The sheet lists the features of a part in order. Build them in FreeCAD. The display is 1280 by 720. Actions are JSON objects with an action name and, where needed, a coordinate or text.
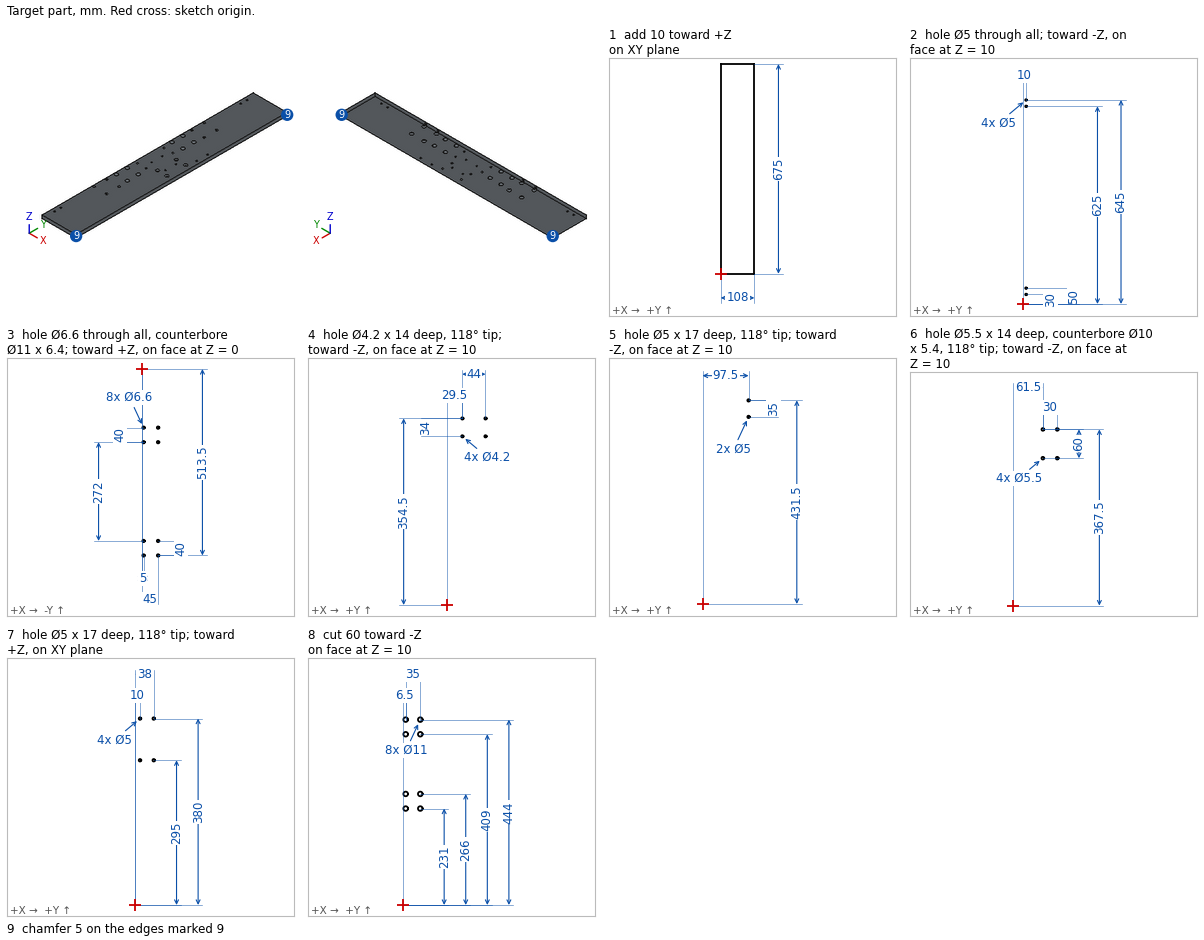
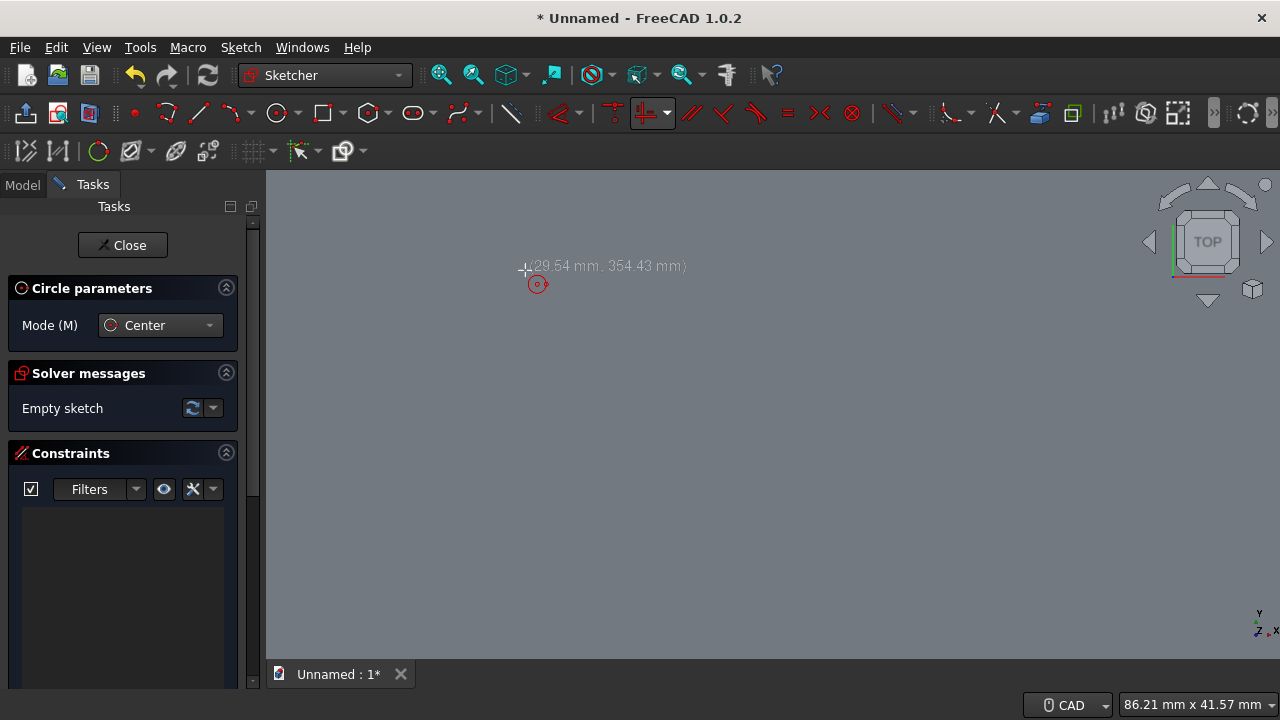
{"action": "left_click", "coordinate": [524, 271]}
{"action": "mouse_move", "coordinate": [542, 253]}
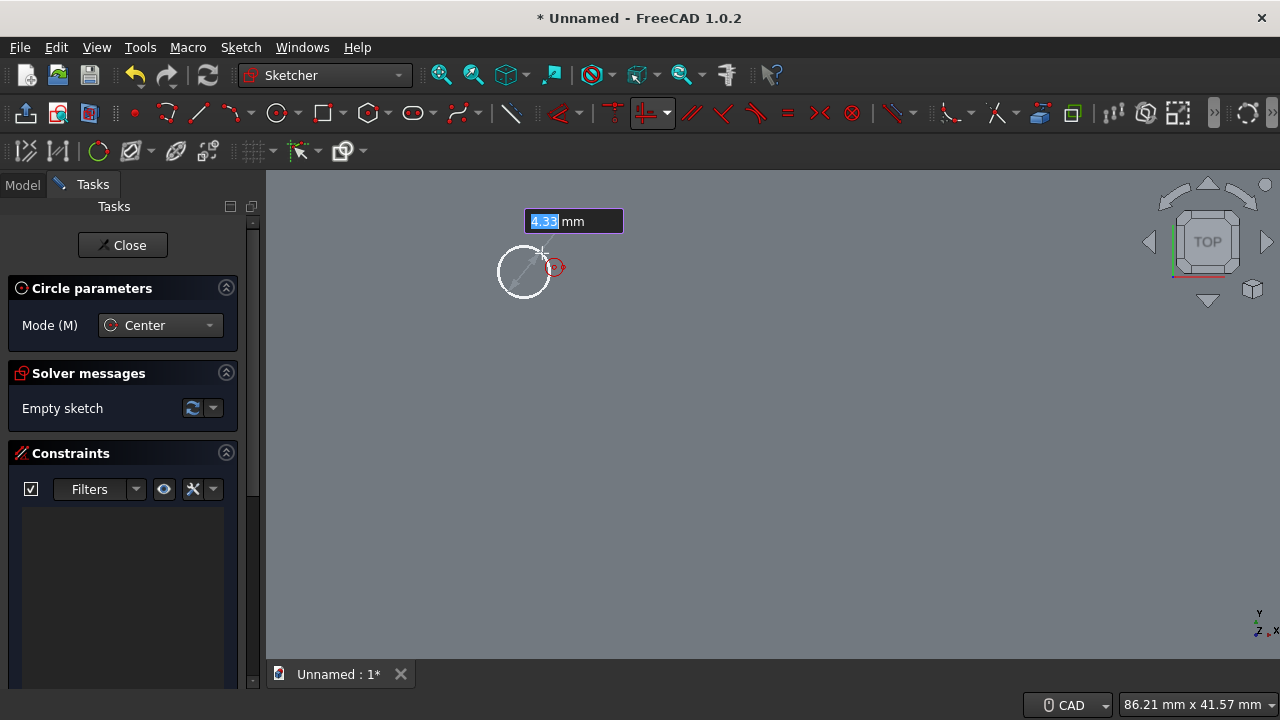
{"action": "type", "text": "4.2"}
{"action": "key", "text": "Return"}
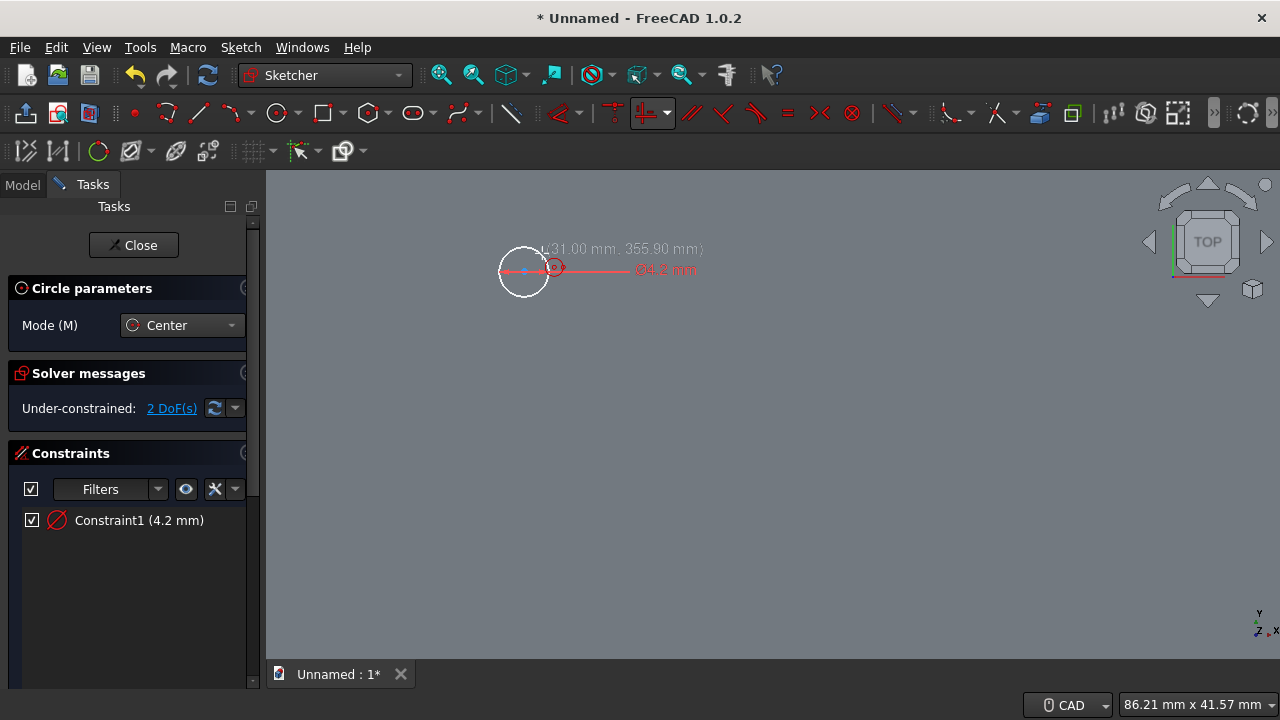
{"action": "left_click", "coordinate": [1042, 271]}
{"action": "mouse_move", "coordinate": [1059, 253]}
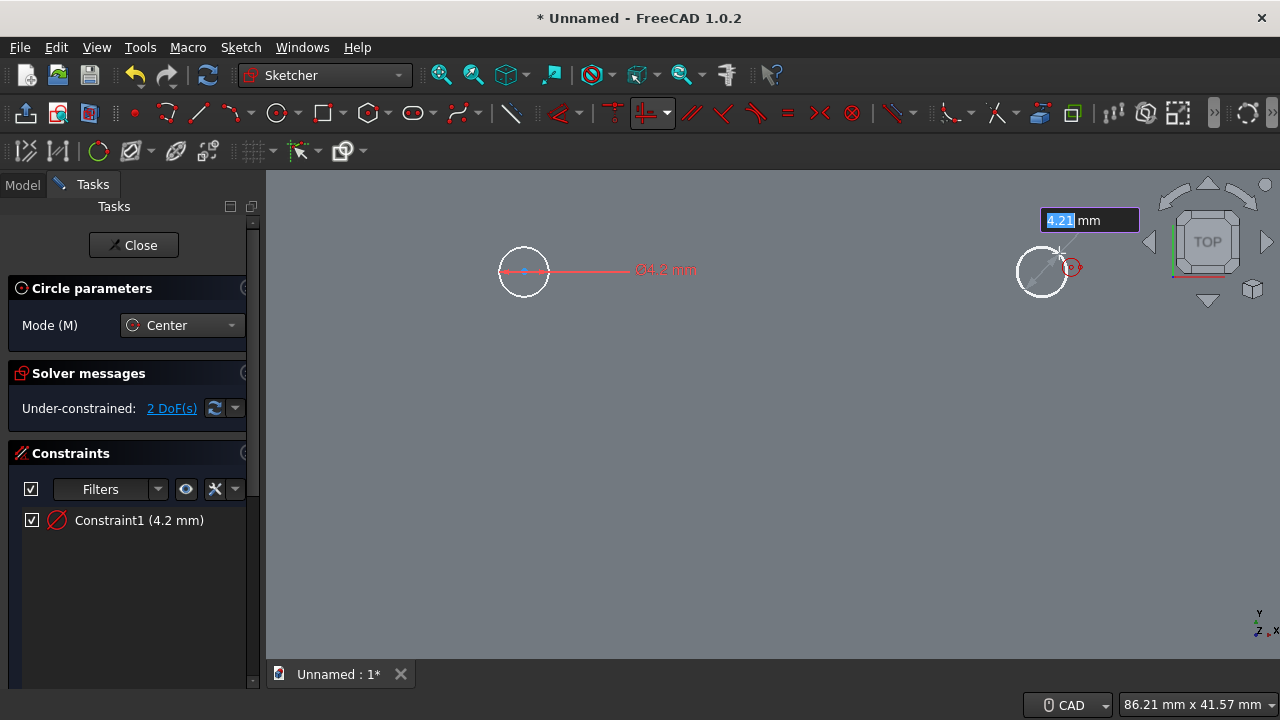
{"action": "type", "text": "4.2"}
{"action": "key", "text": "Return"}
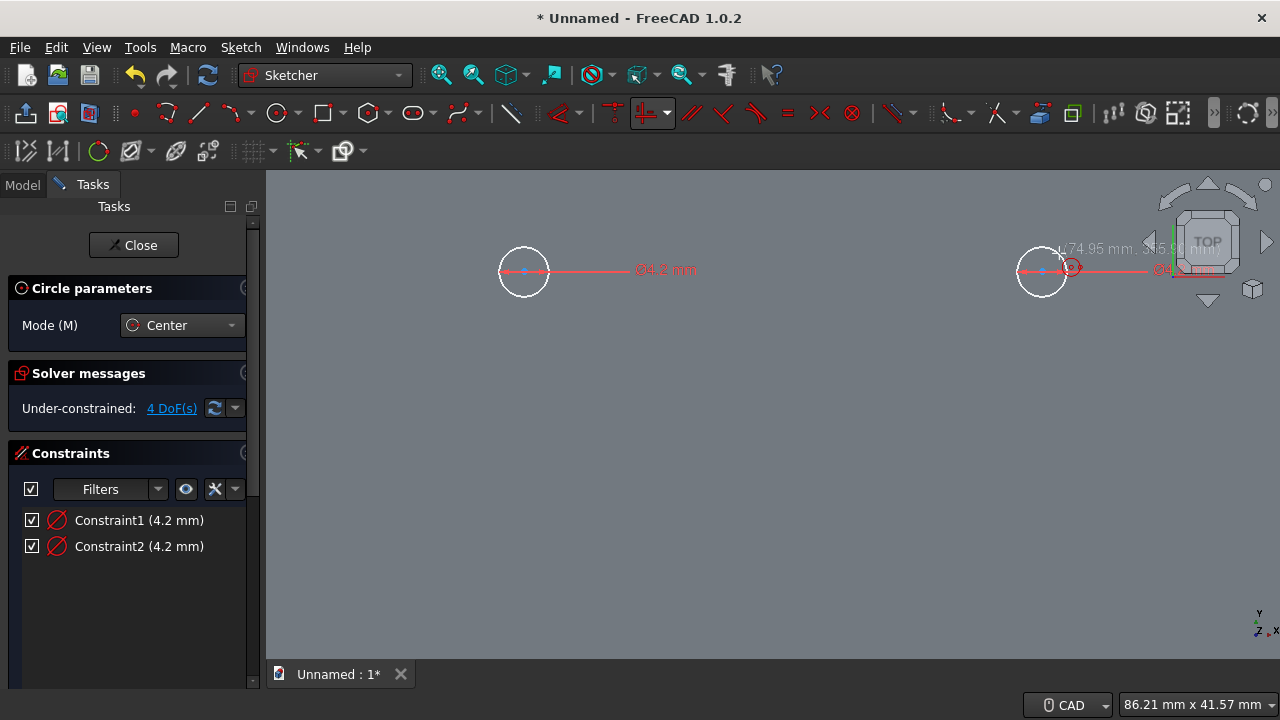
{"action": "scroll", "coordinate": [545, 301], "scroll_direction": "down", "scroll_amount": 2}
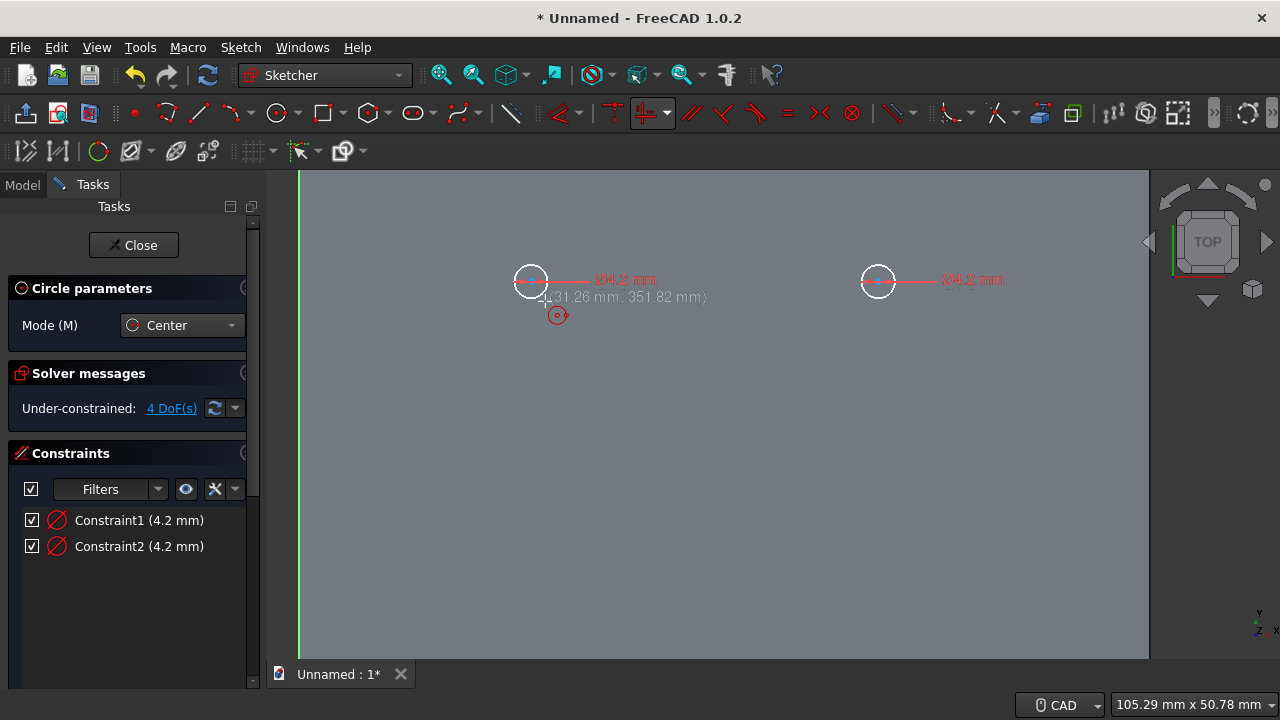
{"action": "scroll", "coordinate": [531, 549], "scroll_direction": "up", "scroll_amount": 2}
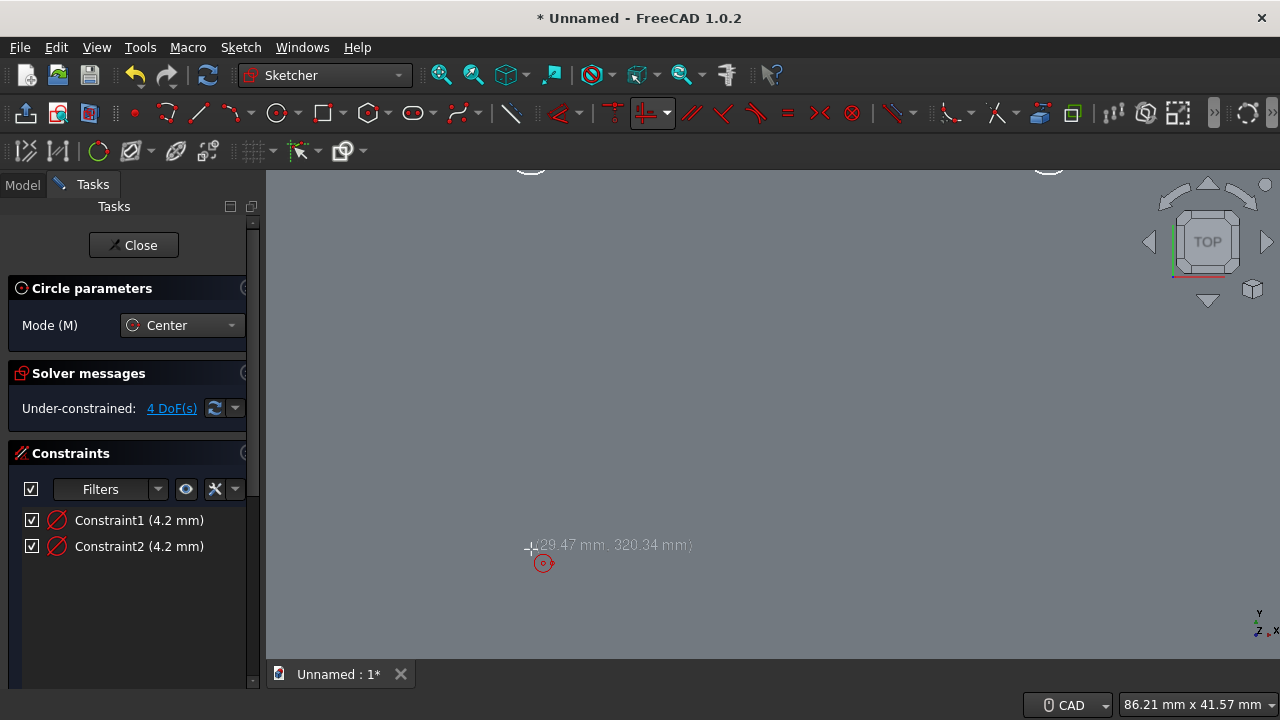
{"action": "left_click", "coordinate": [531, 548]}
{"action": "mouse_move", "coordinate": [549, 531]}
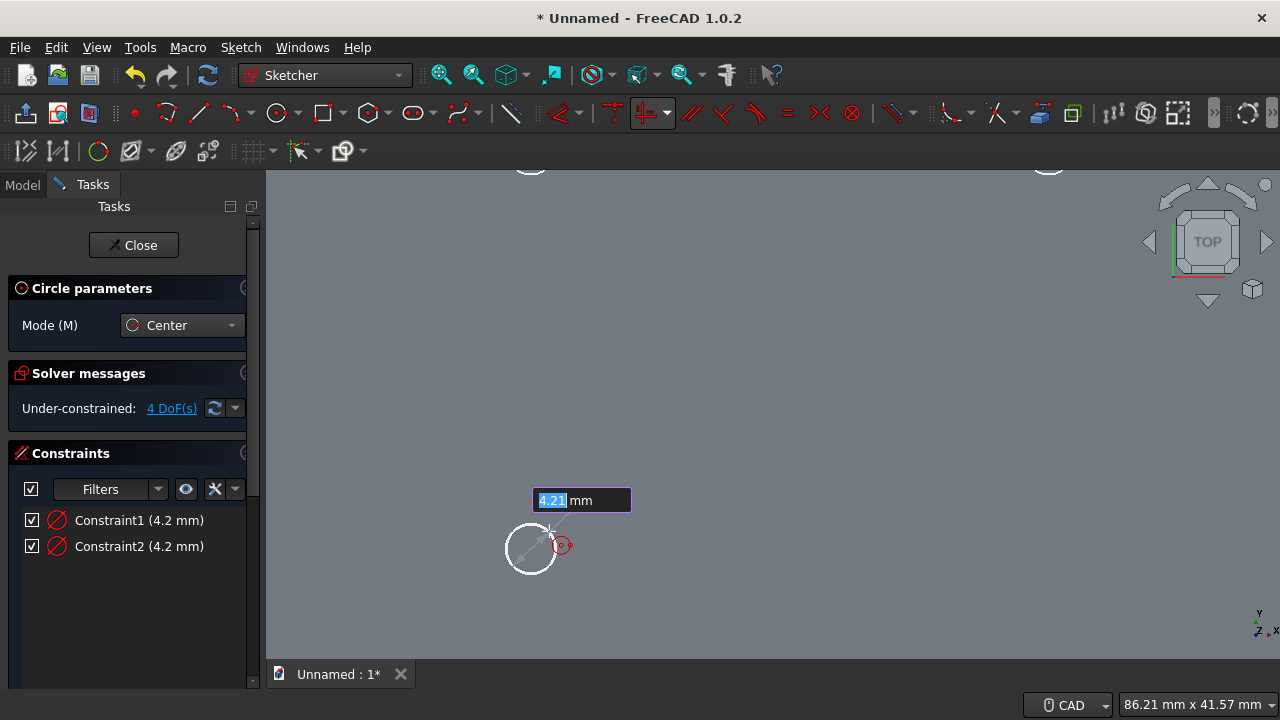
{"action": "type", "text": "4.2"}
{"action": "key", "text": "Return"}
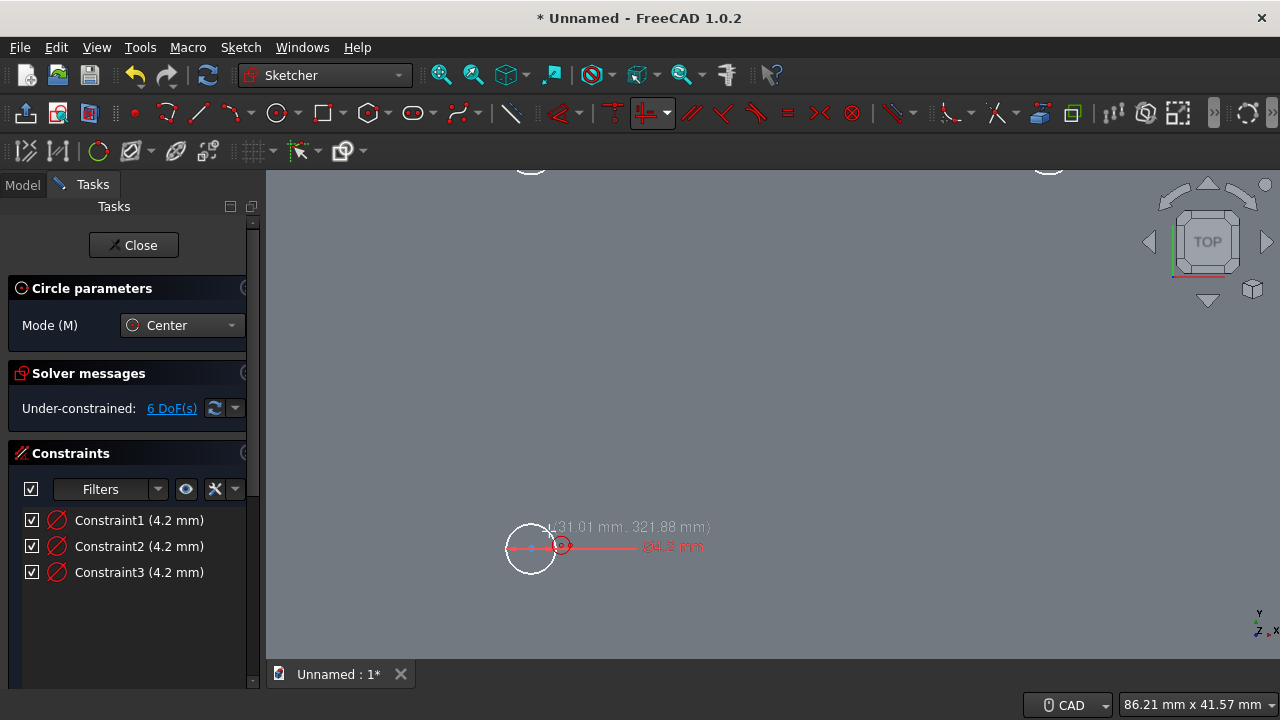
{"action": "left_click", "coordinate": [1049, 548]}
{"action": "mouse_move", "coordinate": [1066, 531]}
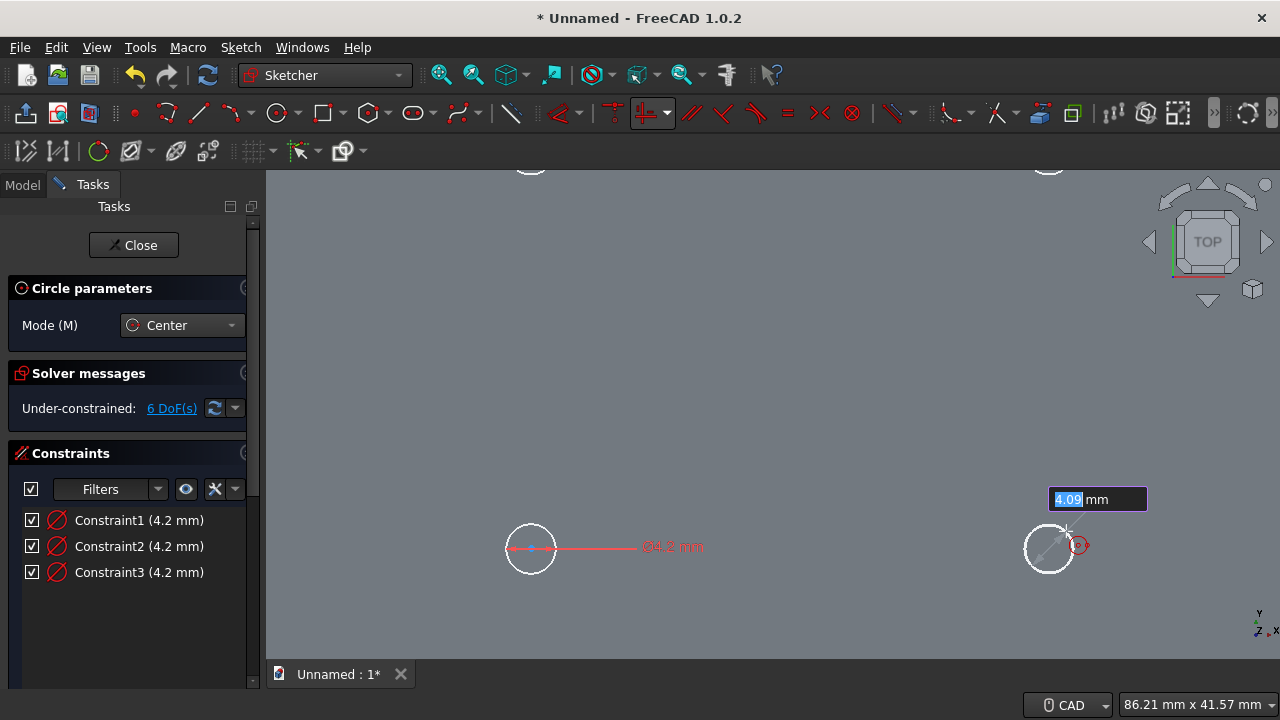
{"action": "type", "text": "4.2"}
{"action": "key", "text": "Return"}
{"action": "key", "text": "Escape"}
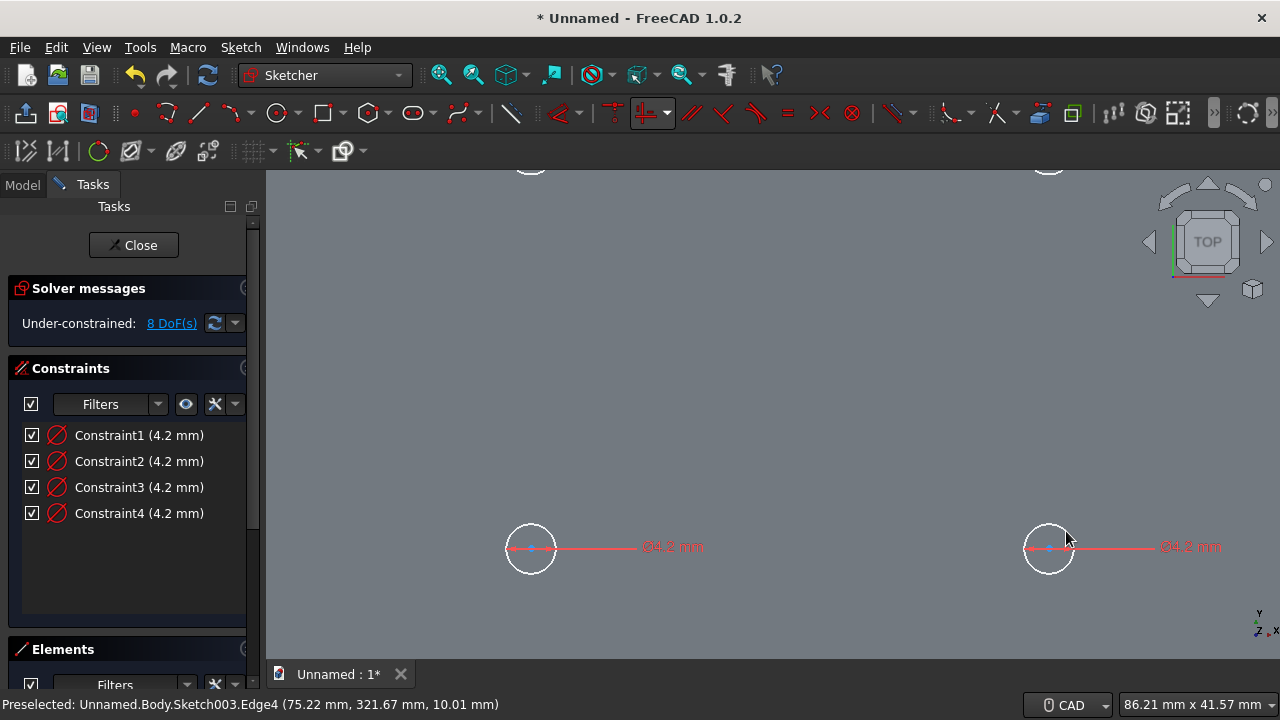
{"action": "scroll", "coordinate": [531, 549], "scroll_direction": "down", "scroll_amount": 2}